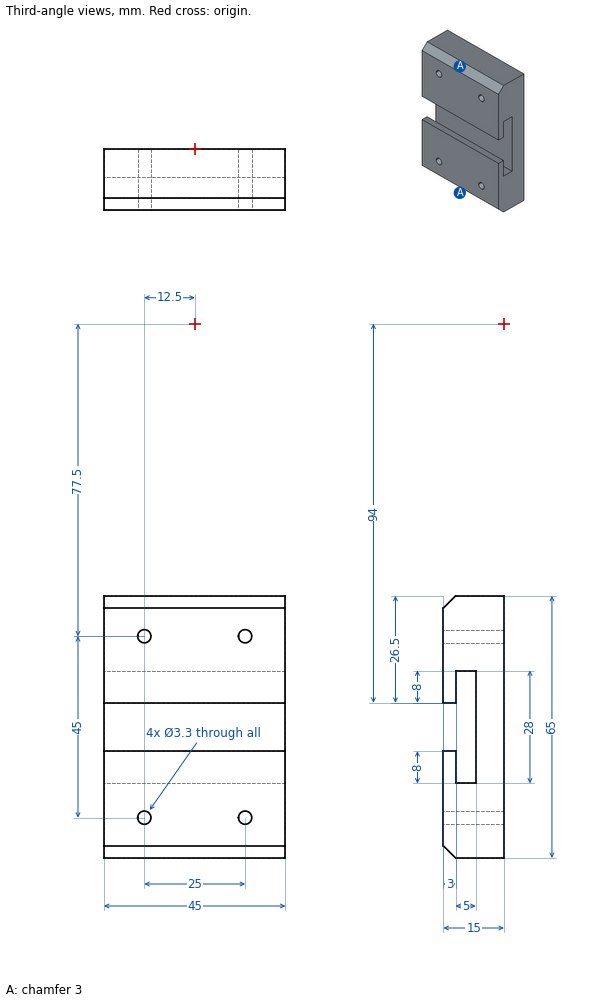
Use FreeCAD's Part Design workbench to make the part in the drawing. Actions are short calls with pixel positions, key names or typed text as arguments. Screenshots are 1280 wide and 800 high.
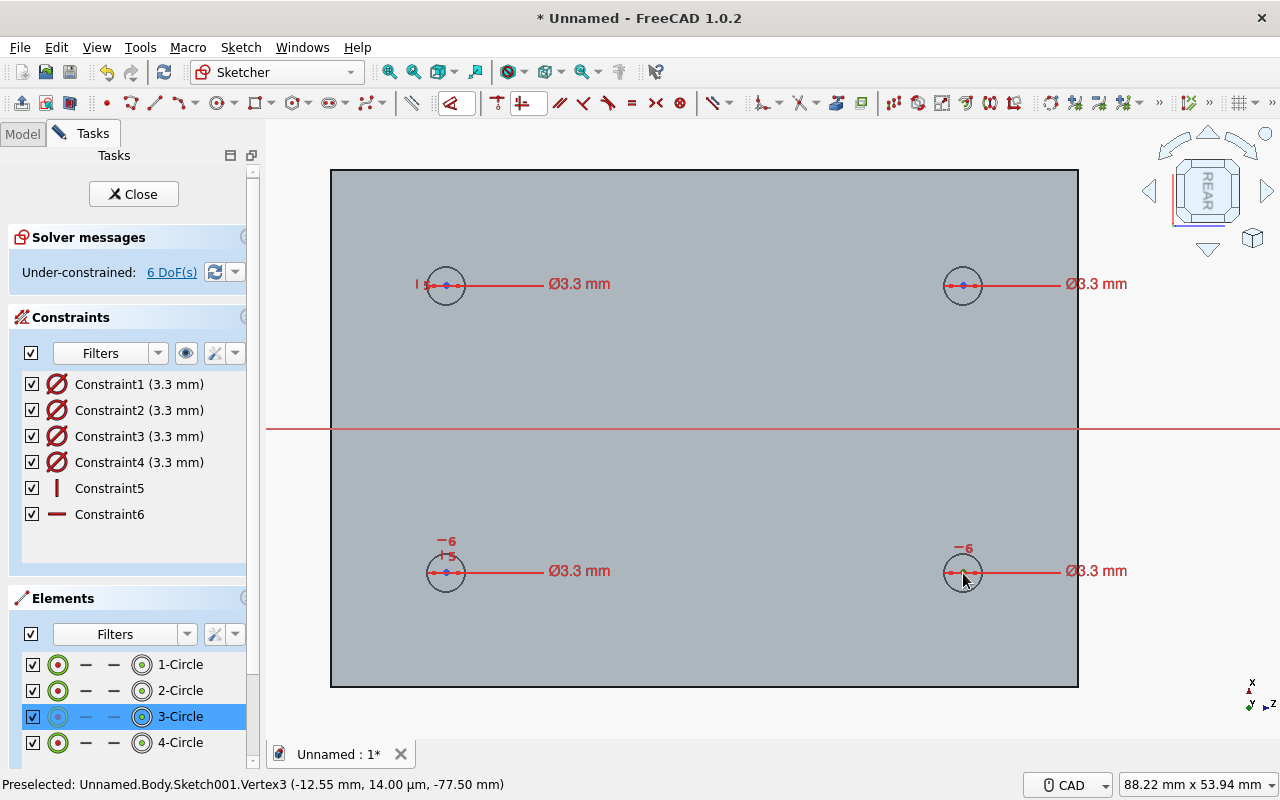
click(963, 286)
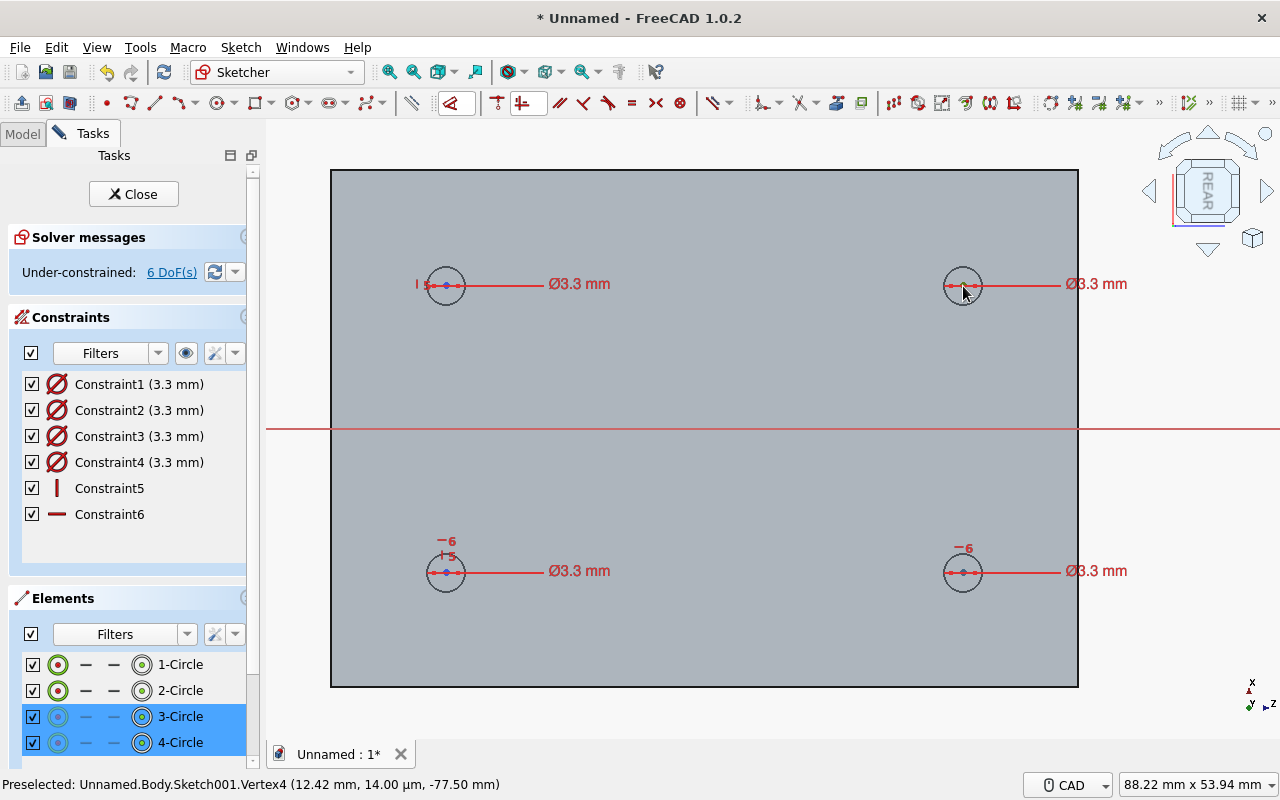
key(v)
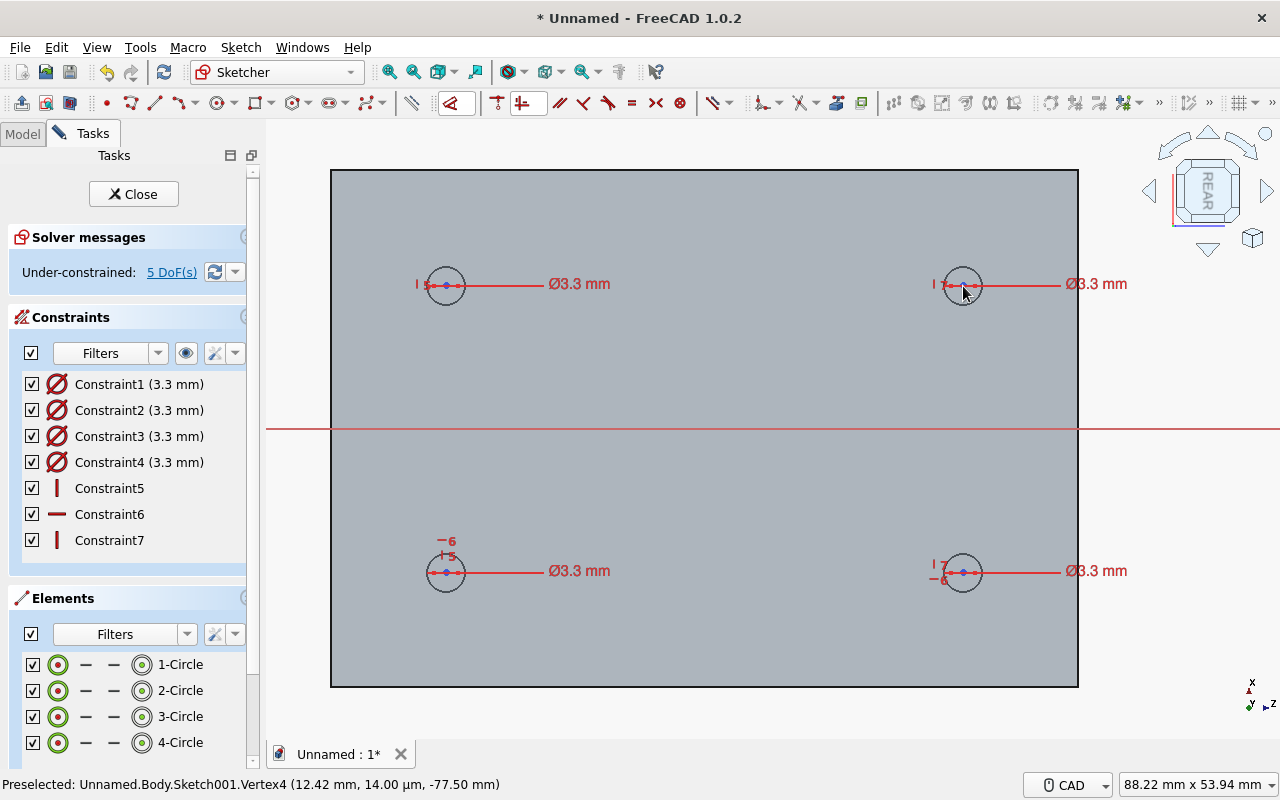
click(446, 286)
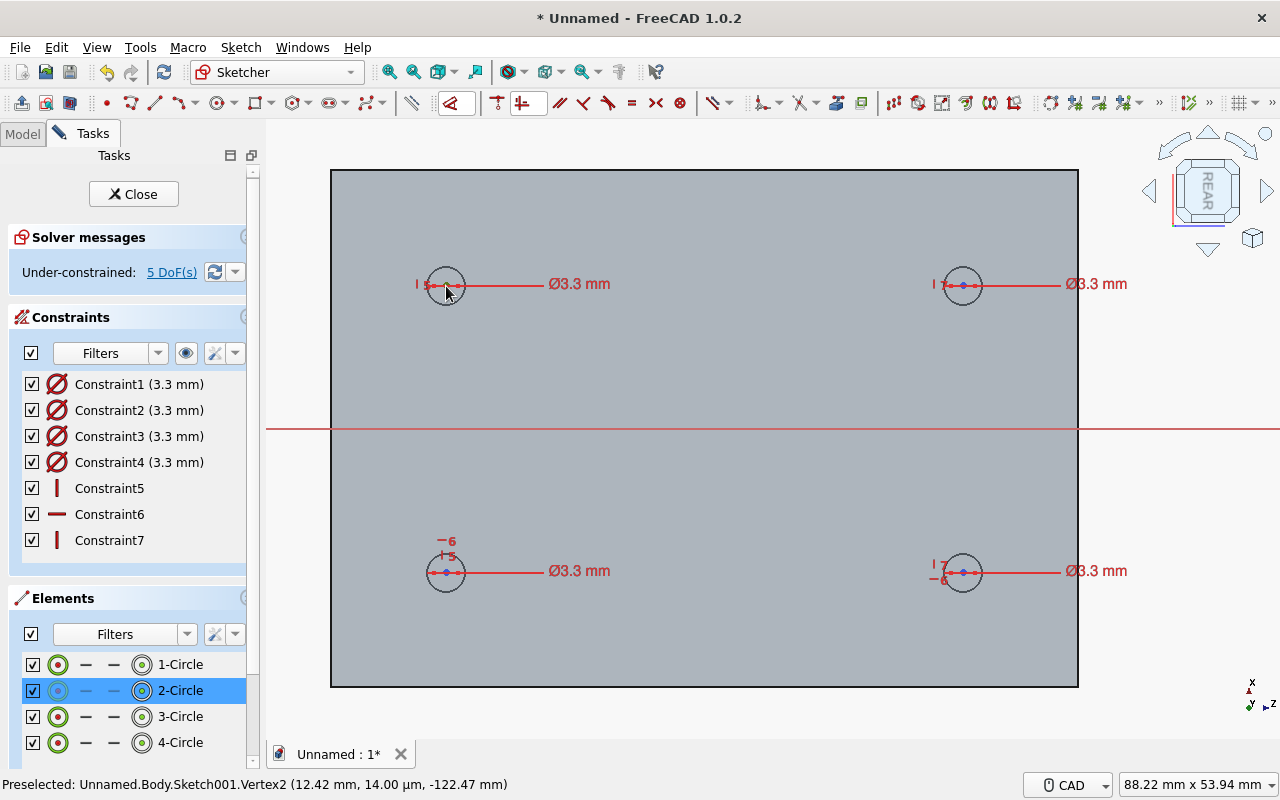
click(963, 286)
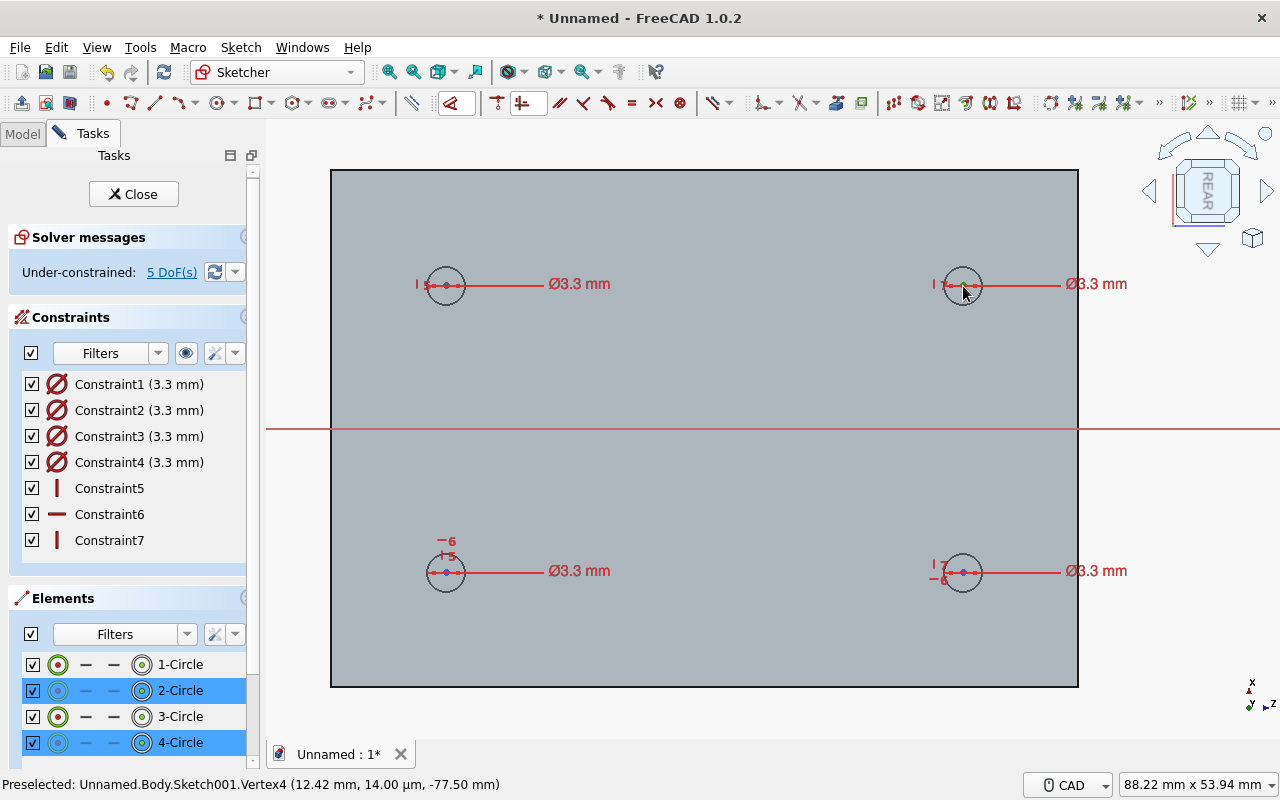
click(542, 104)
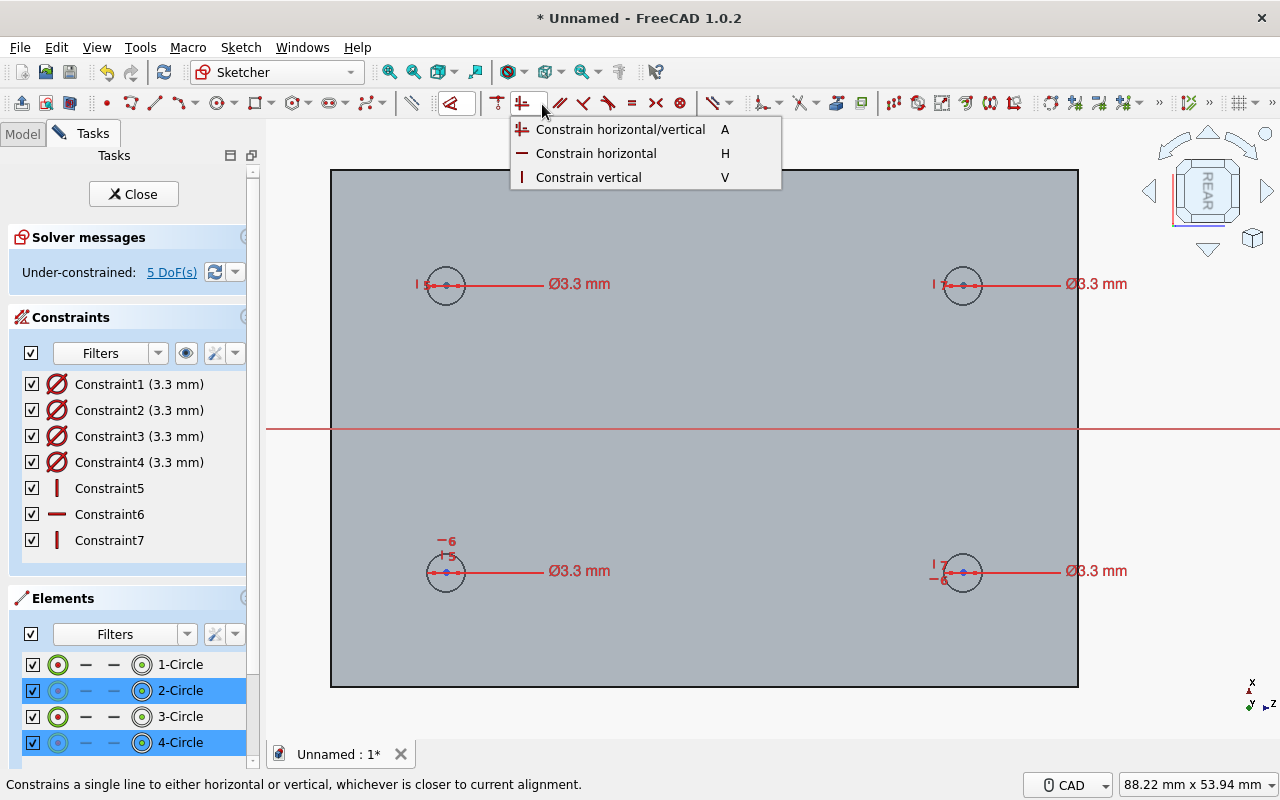
click(646, 153)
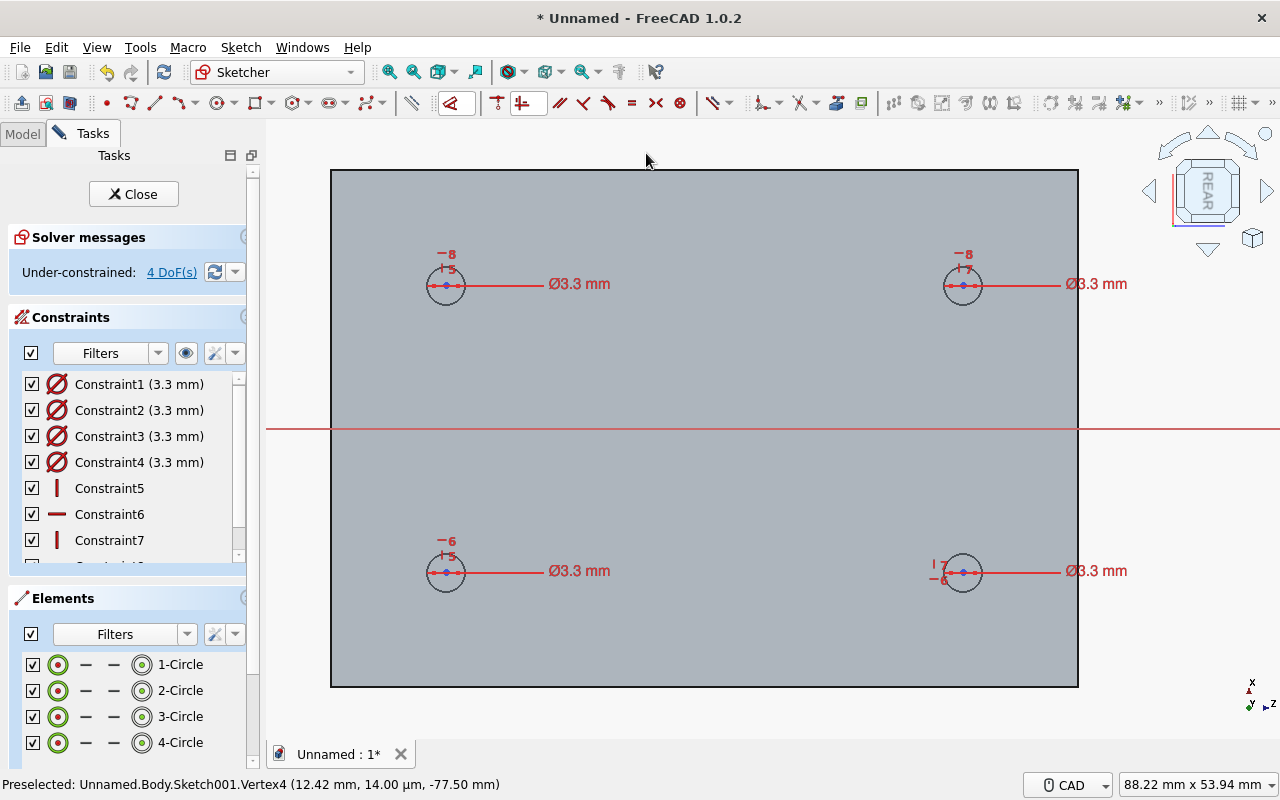
click(446, 573)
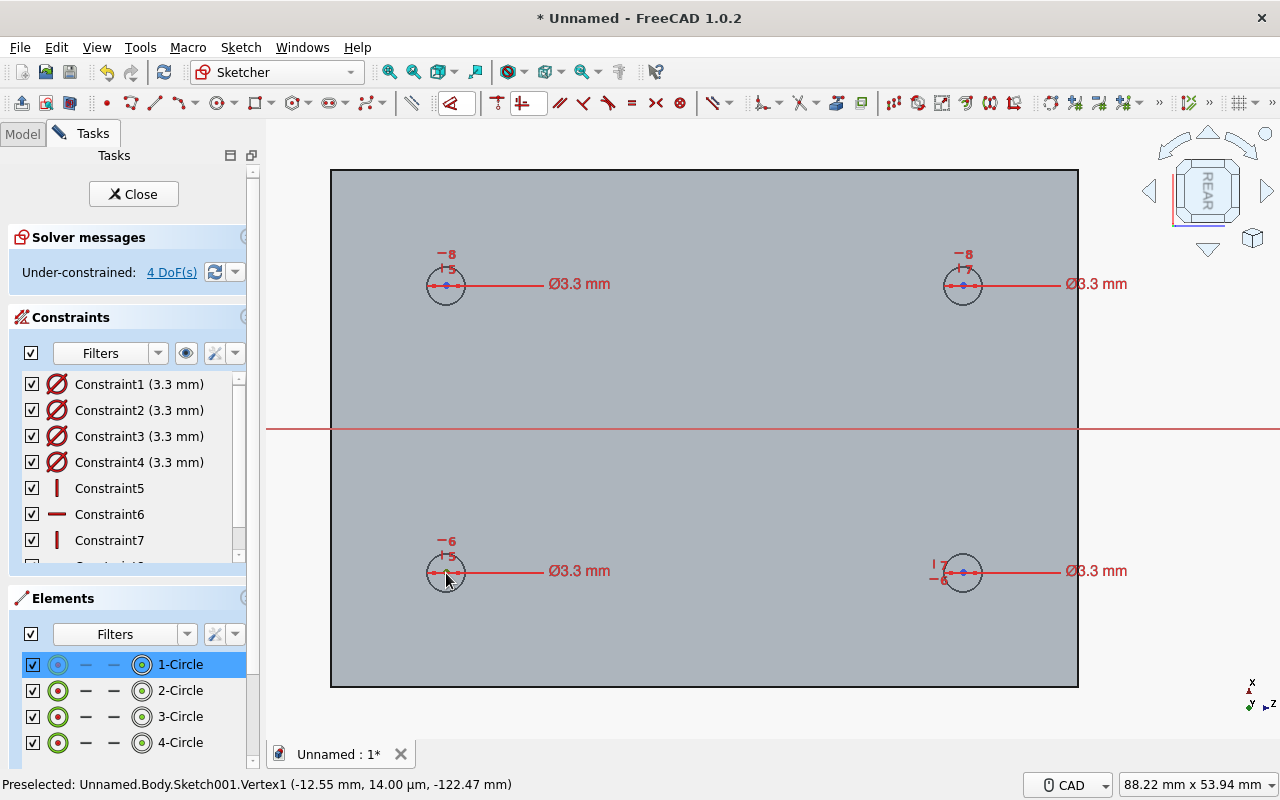
click(446, 286)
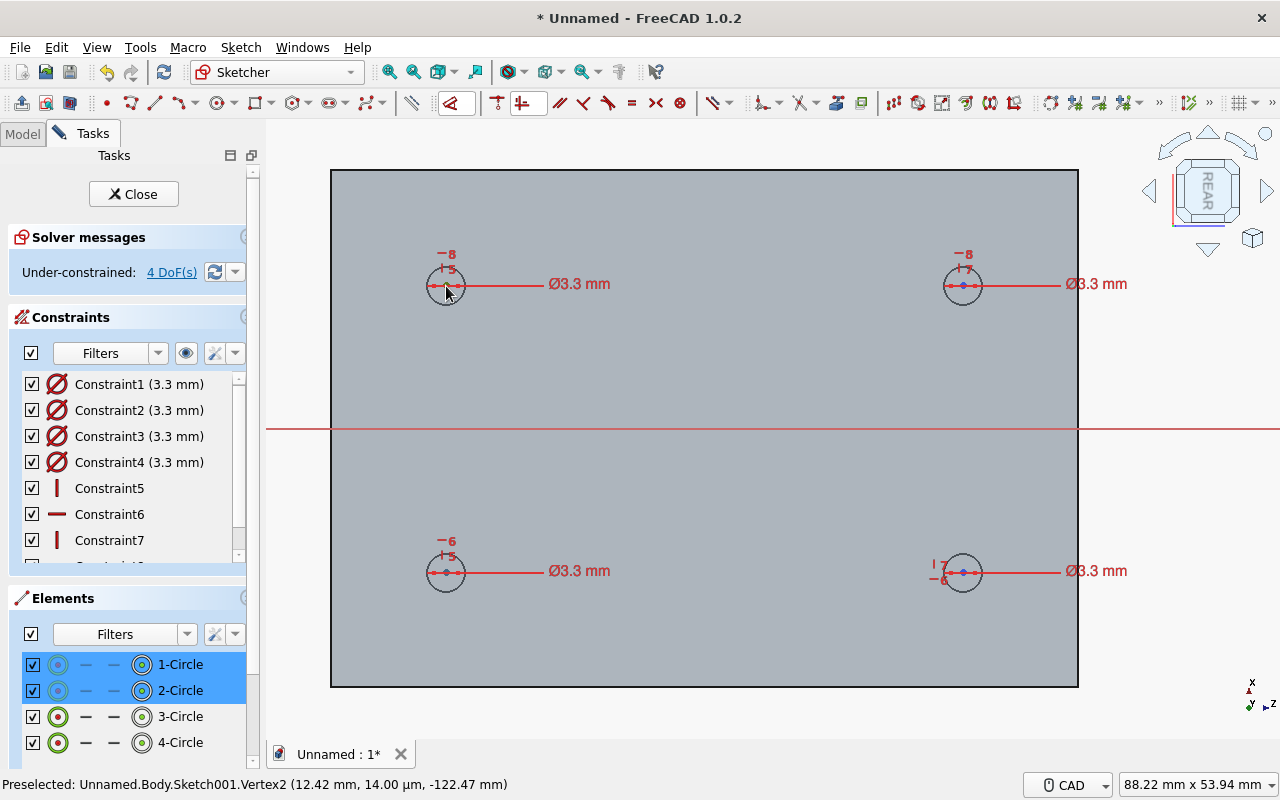
click(470, 104)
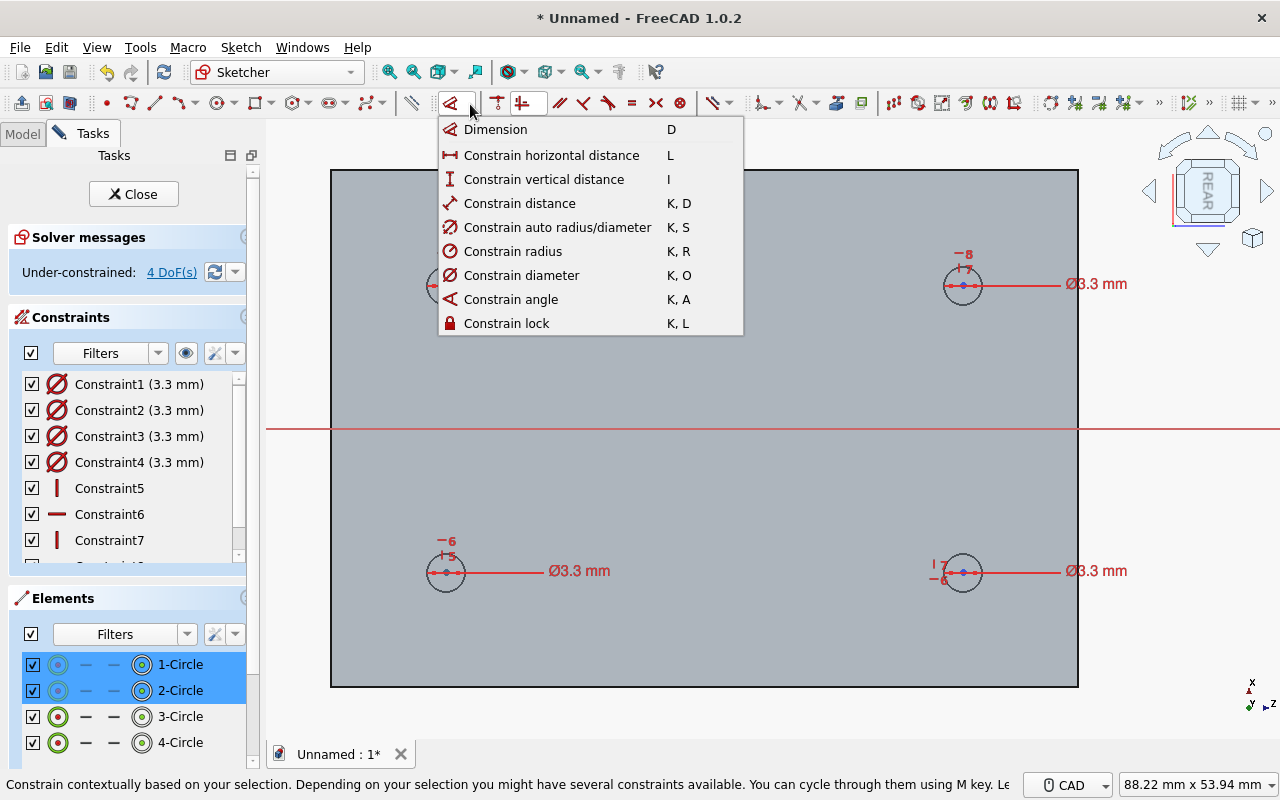
click(591, 179)